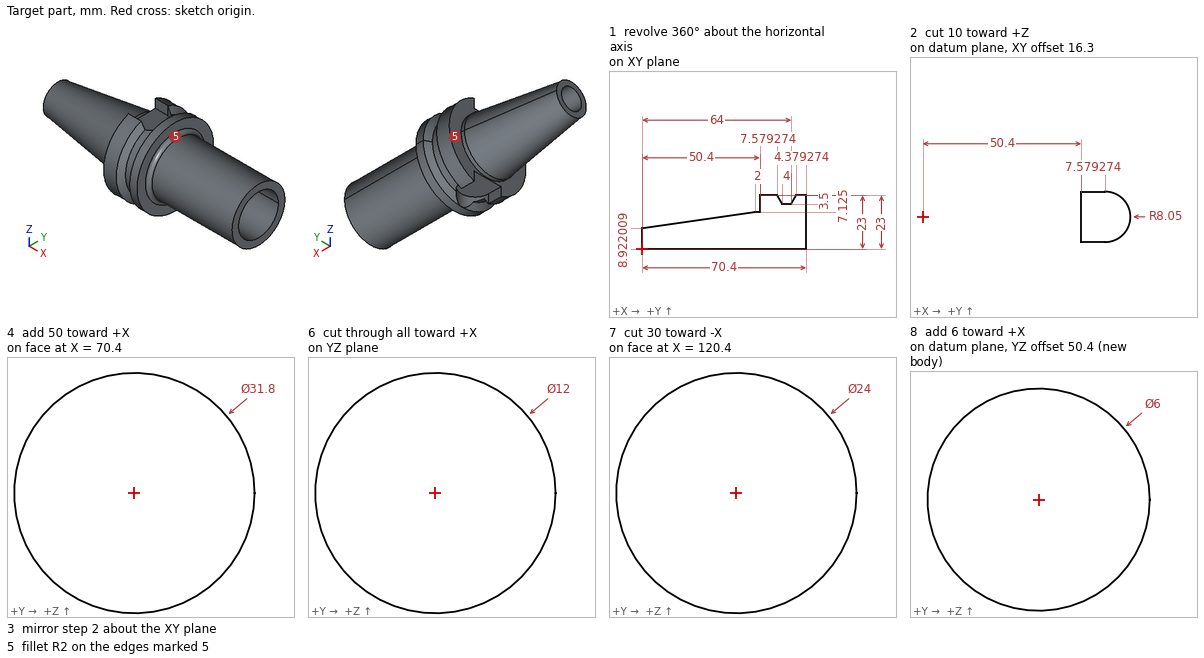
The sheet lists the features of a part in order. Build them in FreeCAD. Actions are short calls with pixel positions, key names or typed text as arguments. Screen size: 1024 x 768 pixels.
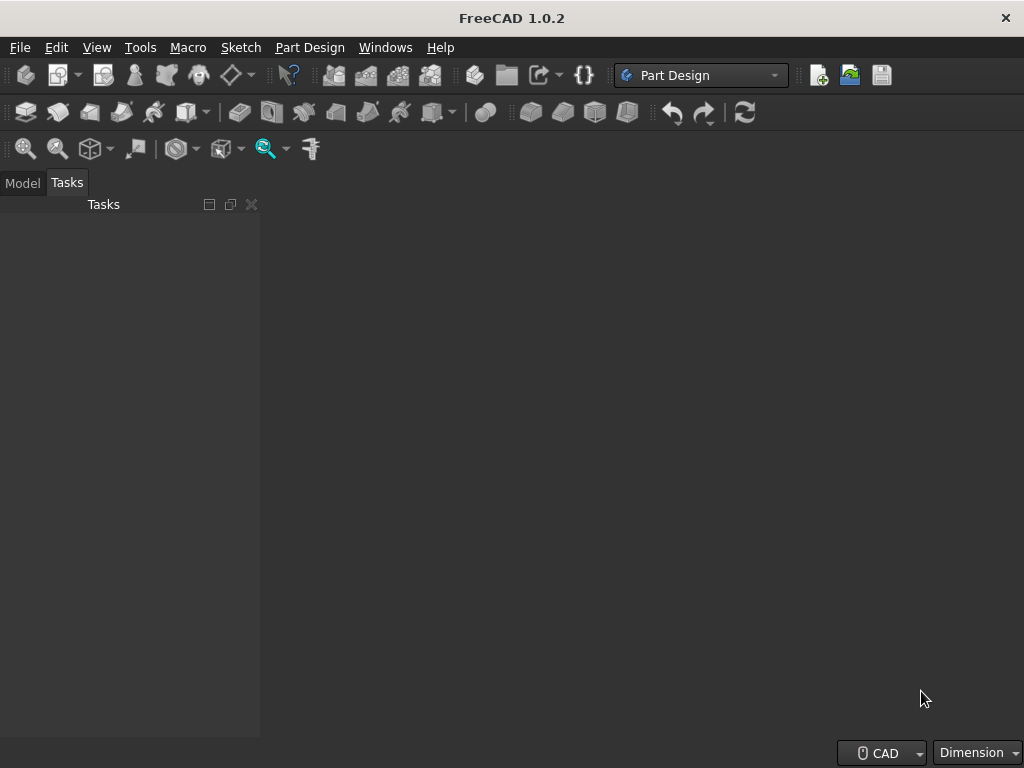
key(ctrl+n)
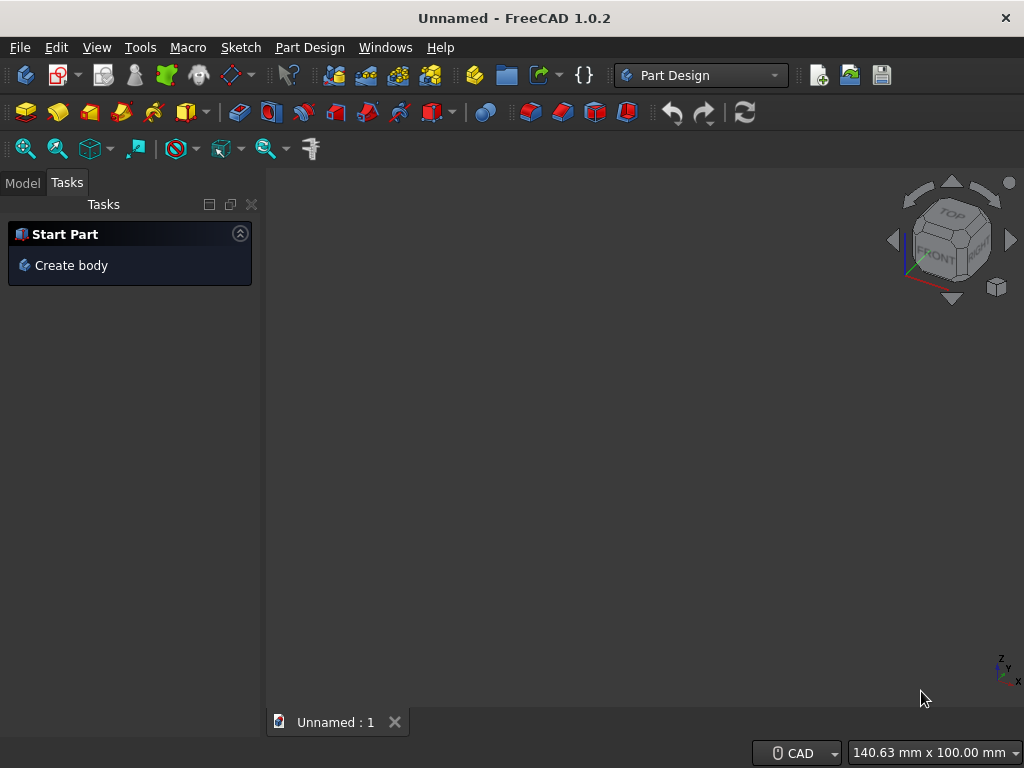
click(58, 76)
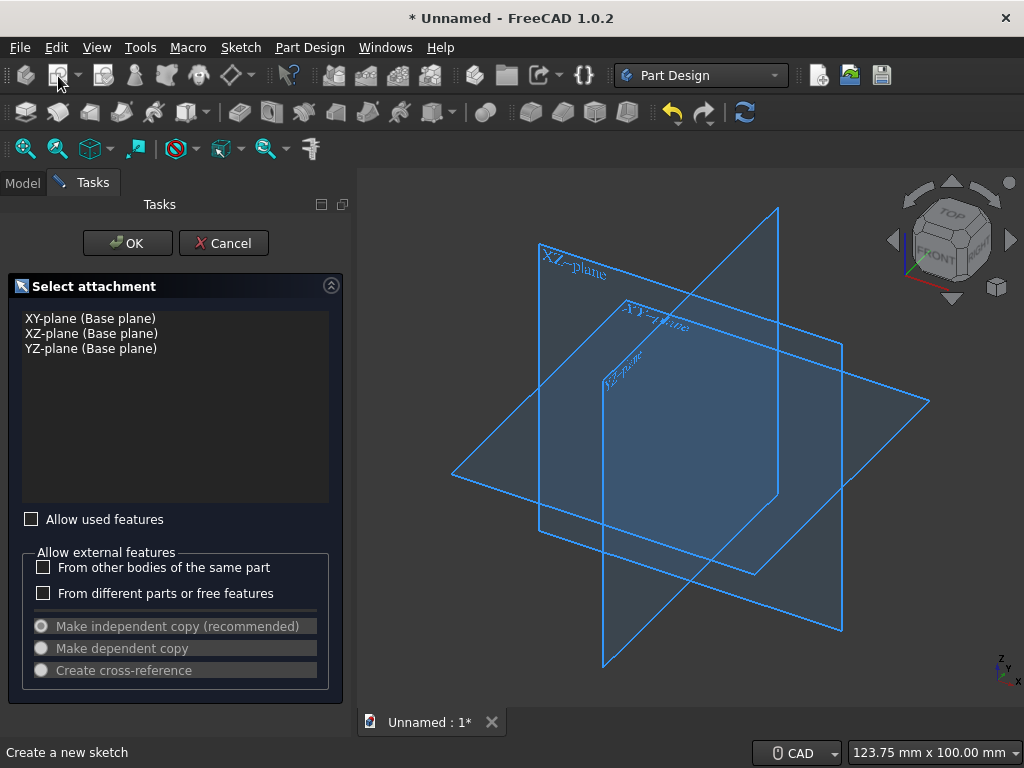
click(82, 318)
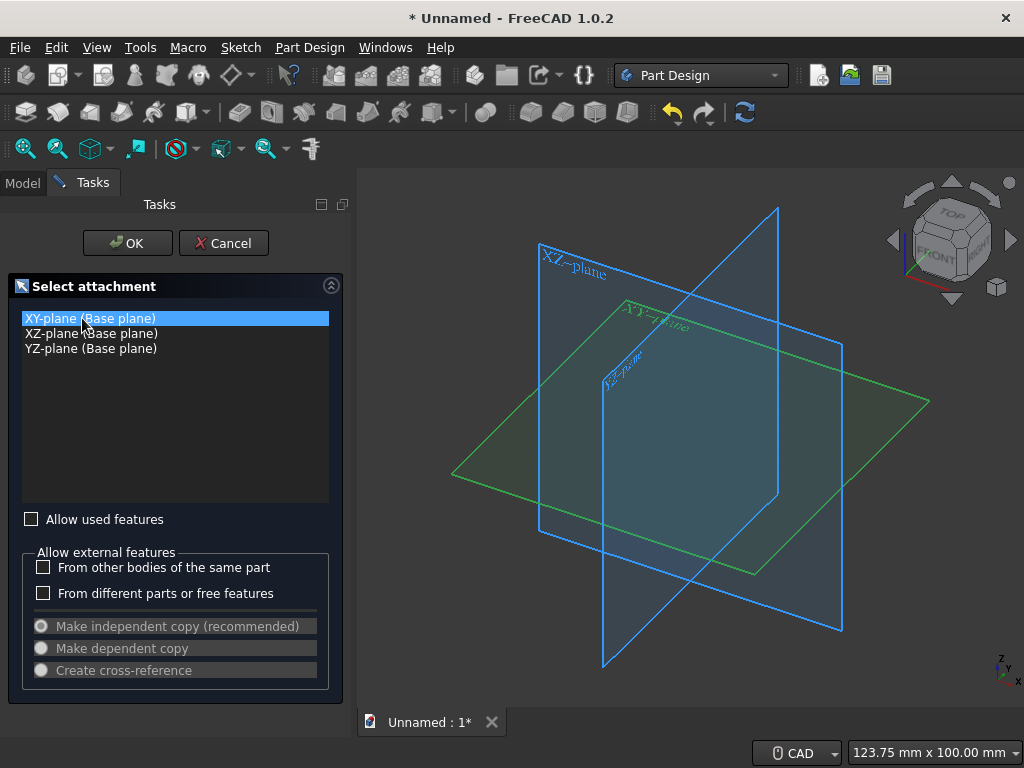
click(128, 243)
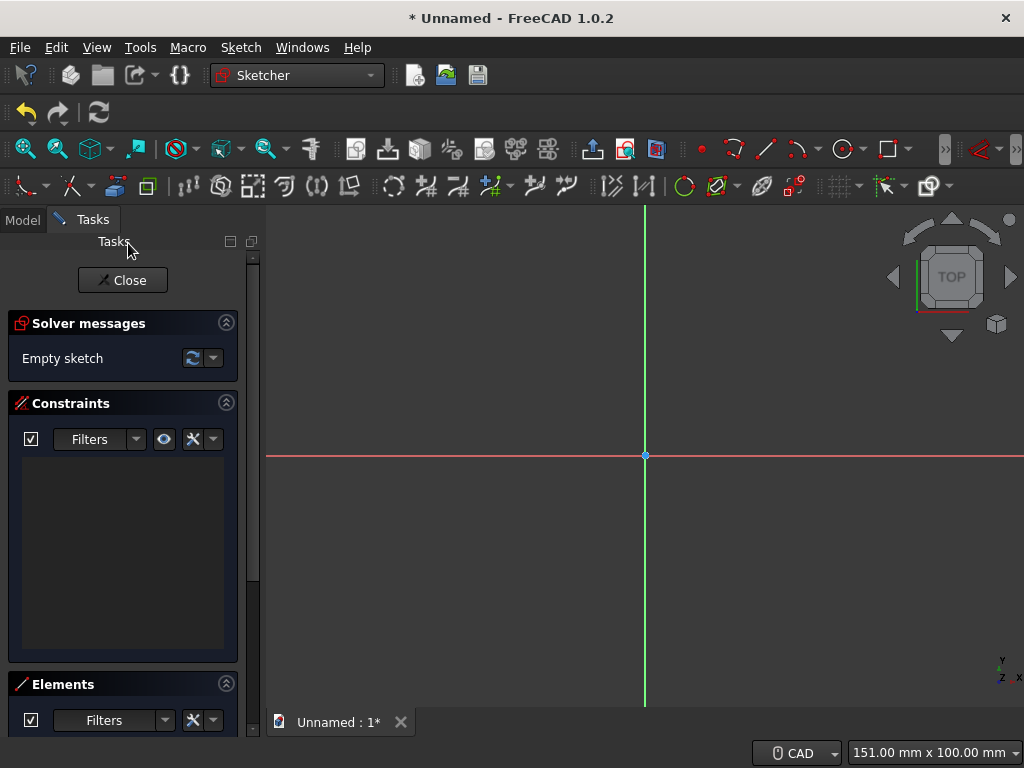
scroll(294, 573, down, 2)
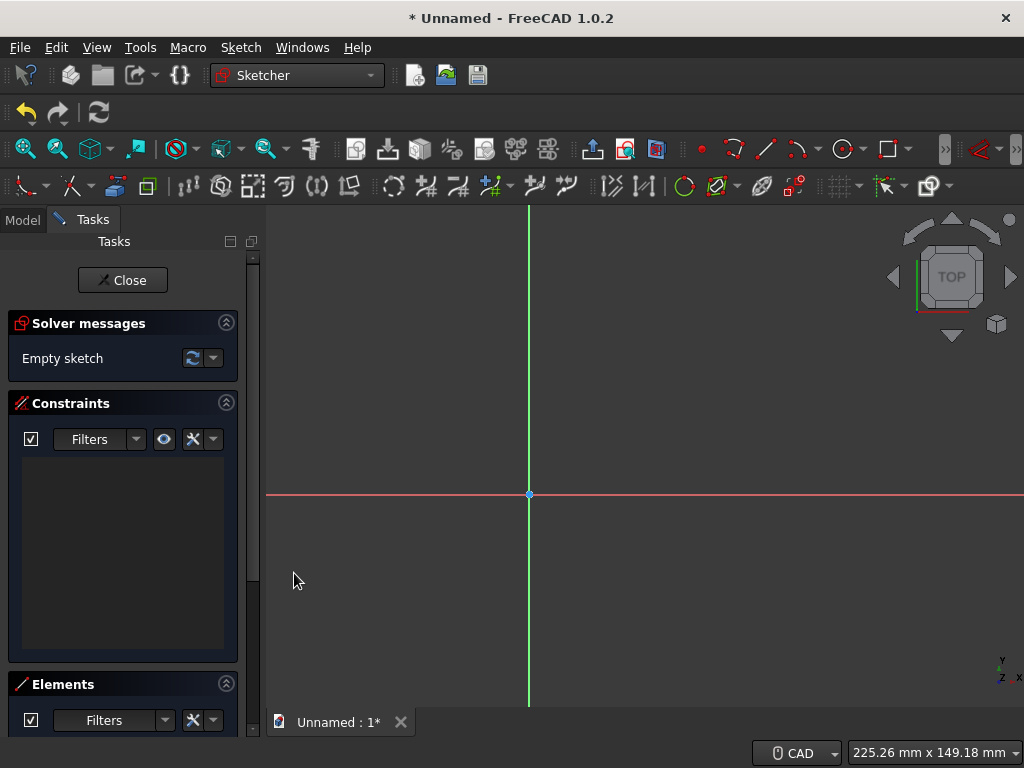
scroll(734, 456, up, 3)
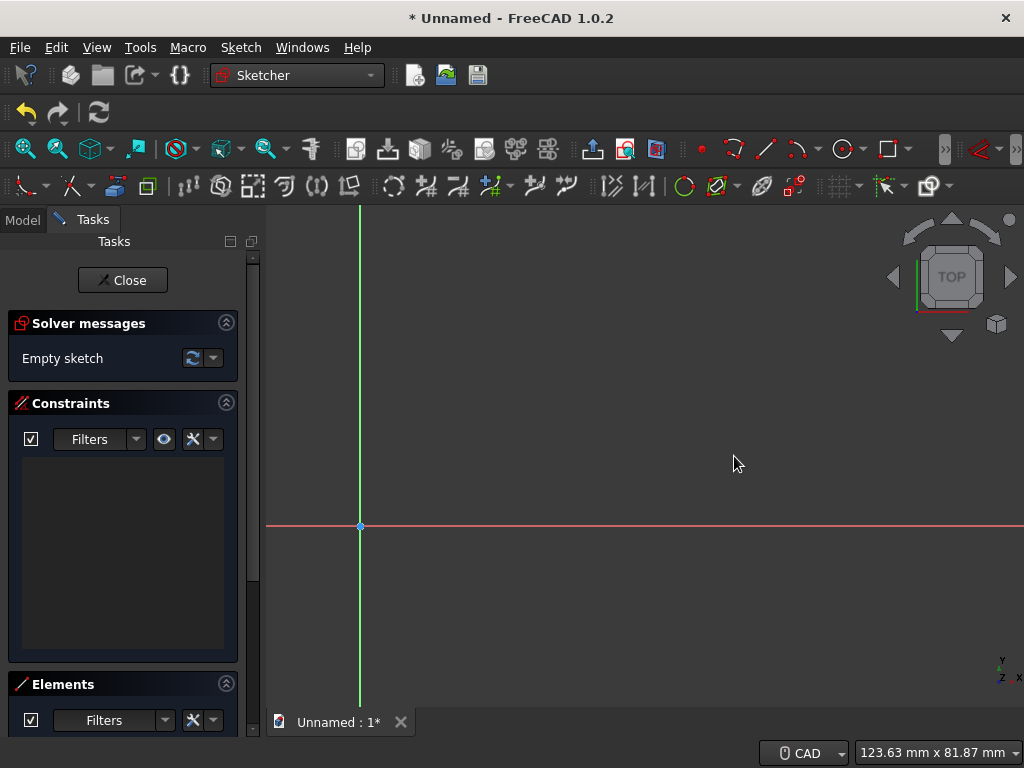
click(734, 150)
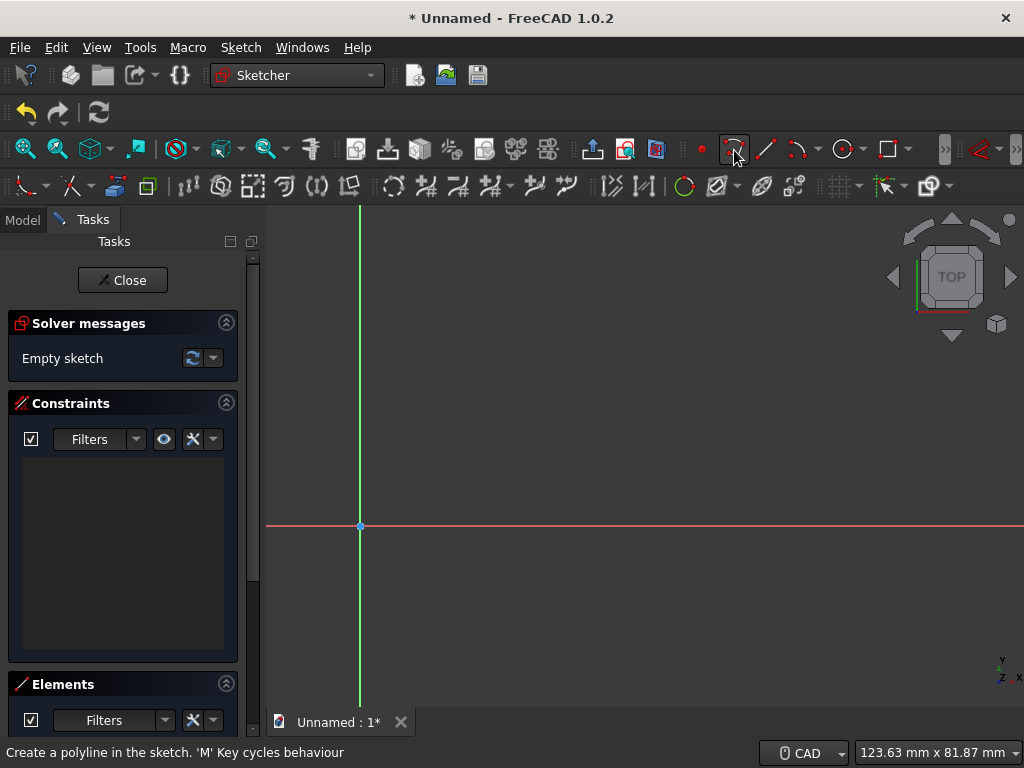
click(360, 526)
click(792, 517)
click(792, 385)
click(765, 385)
click(753, 407)
click(728, 407)
click(716, 385)
click(670, 385)
click(670, 429)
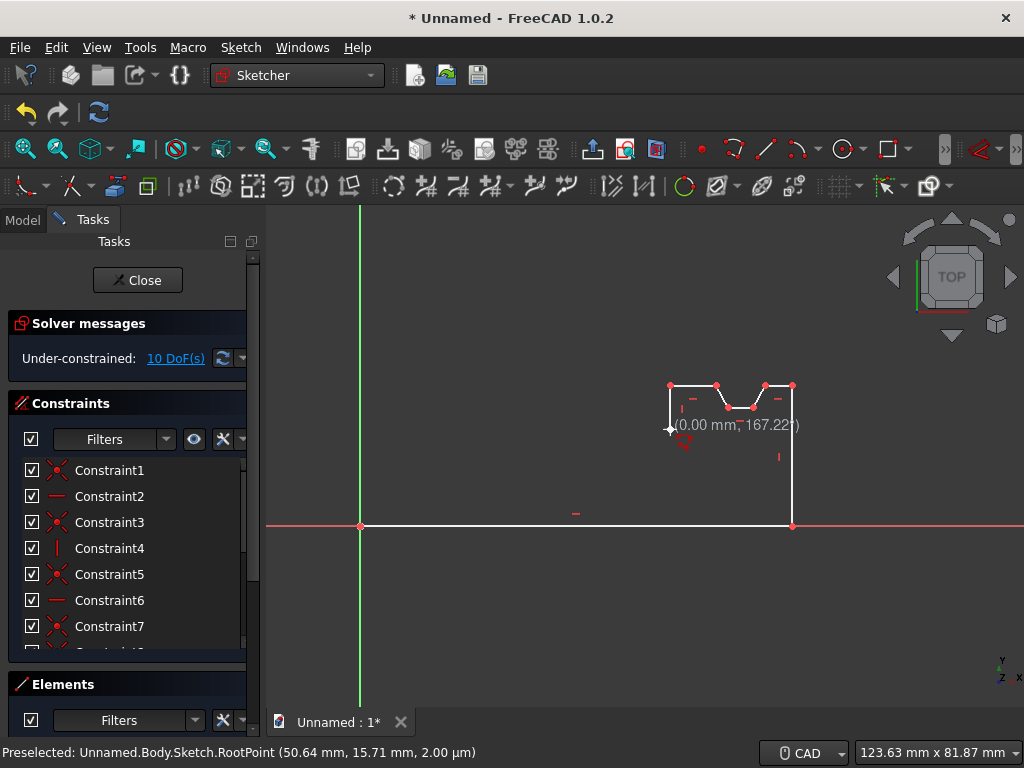
scroll(657, 429, up, 2)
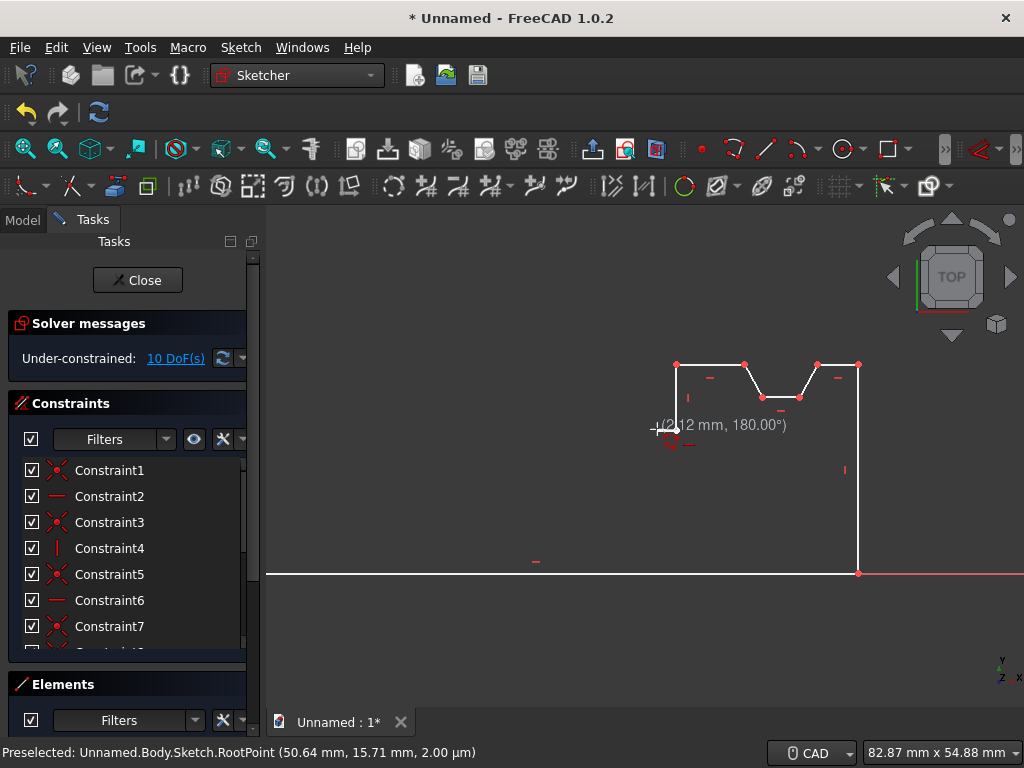
click(657, 429)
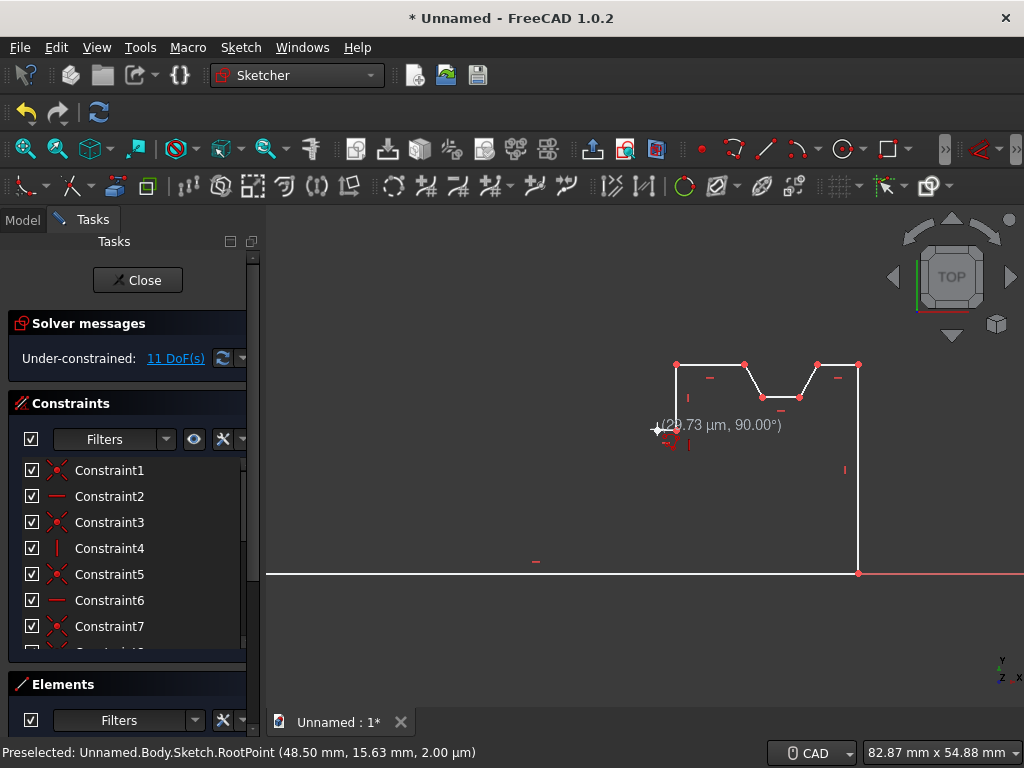
scroll(658, 430, down, 2)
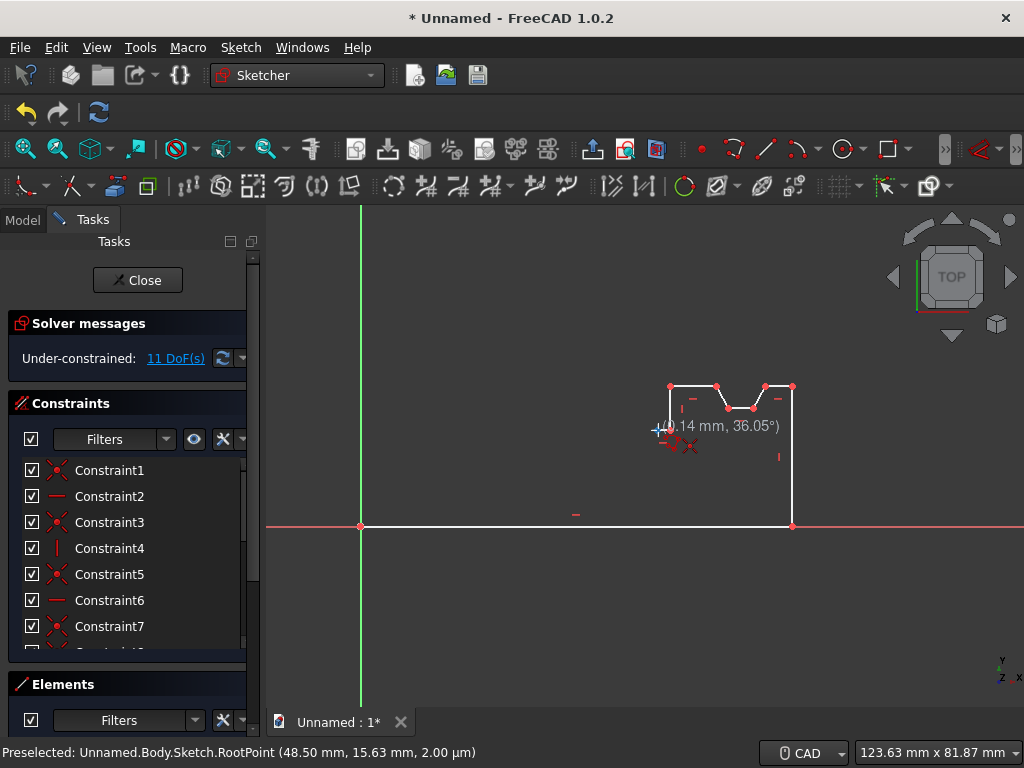
click(370, 472)
click(361, 527)
key(Escape)
key(Escape)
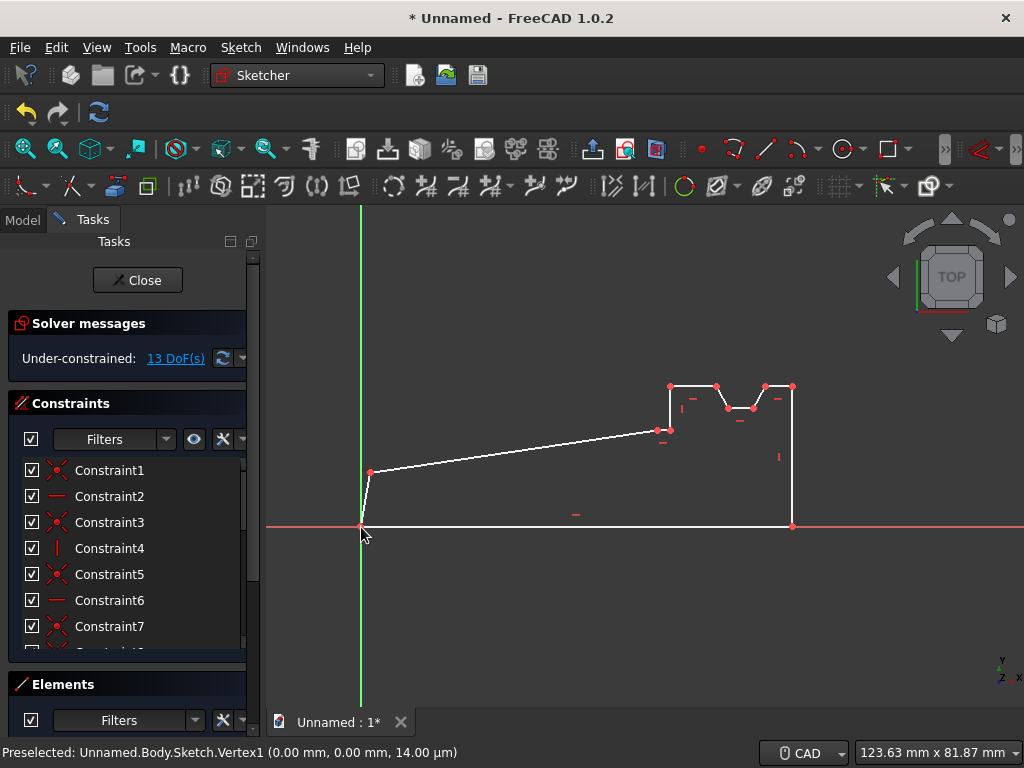
click(364, 511)